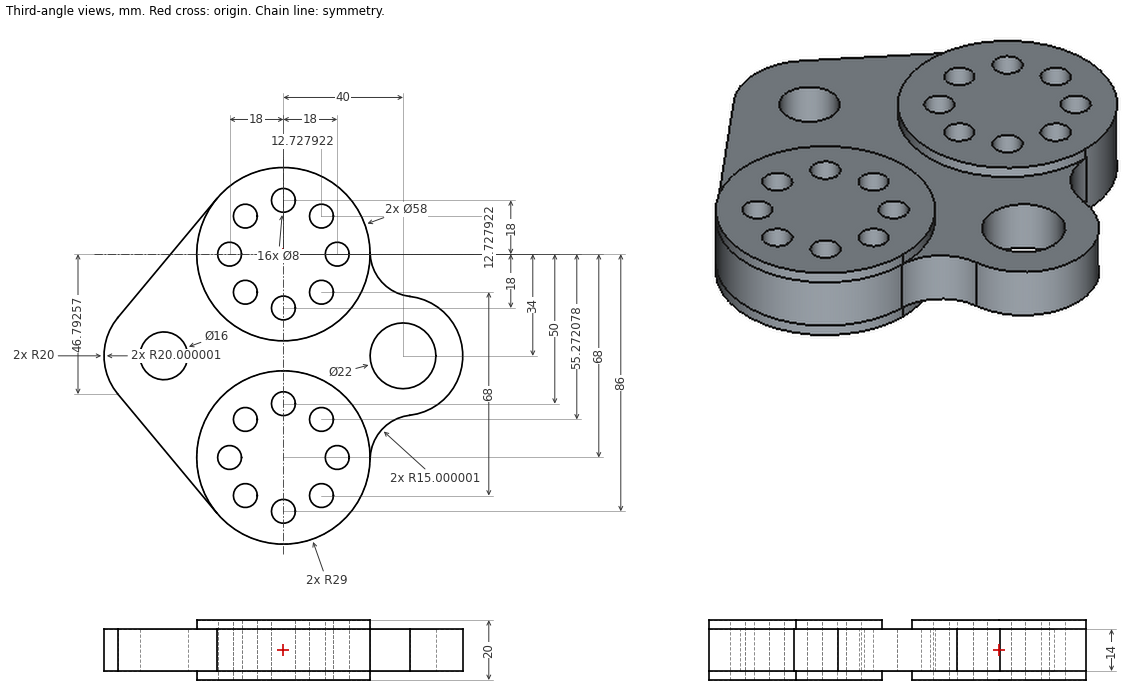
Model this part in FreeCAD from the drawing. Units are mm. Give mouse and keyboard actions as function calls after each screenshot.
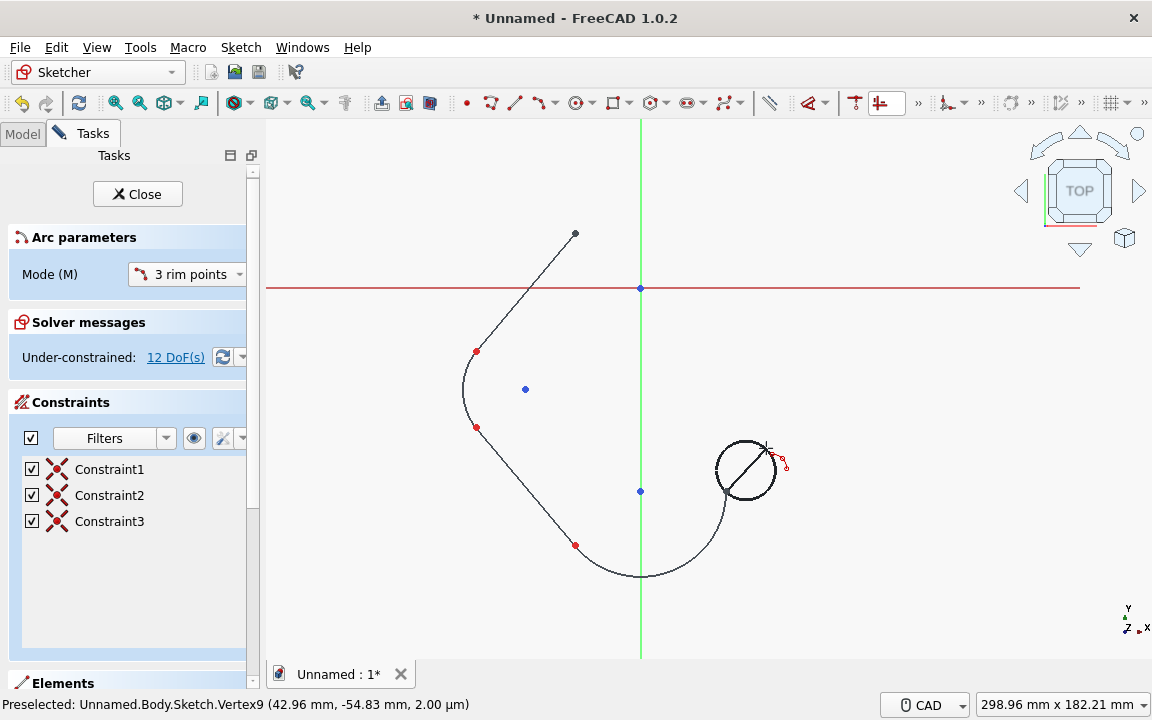
scroll(738, 462, up, 2)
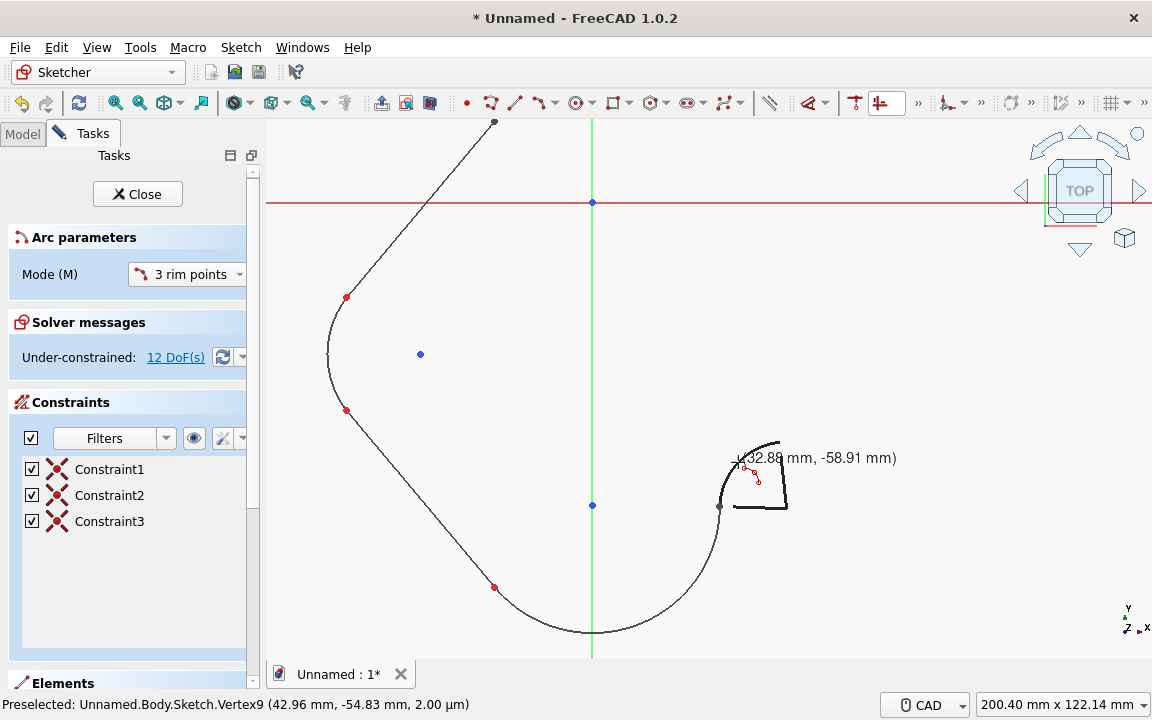
click(738, 462)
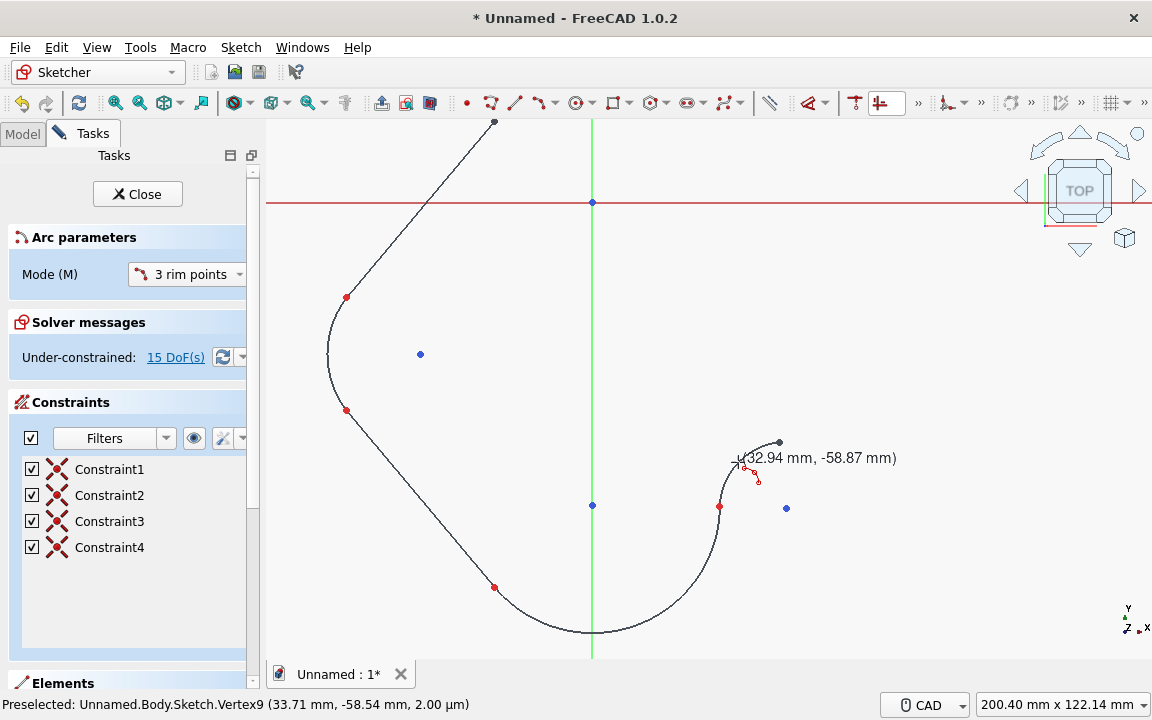
click(780, 442)
click(779, 265)
click(858, 353)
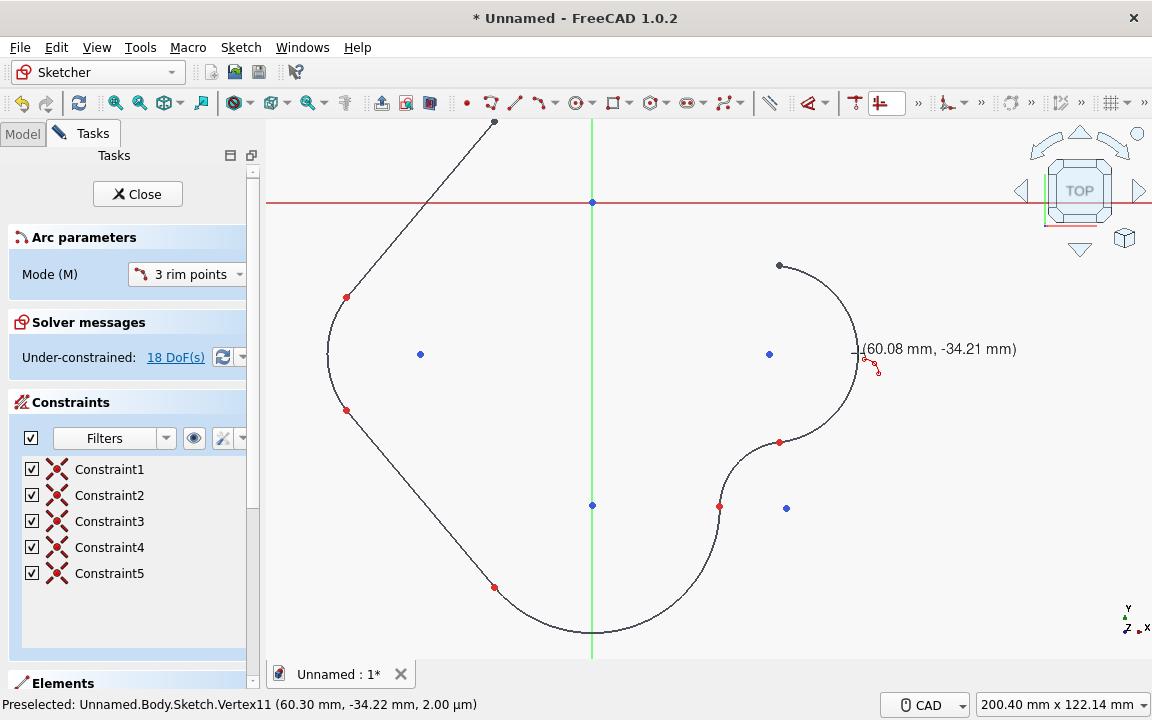
click(779, 266)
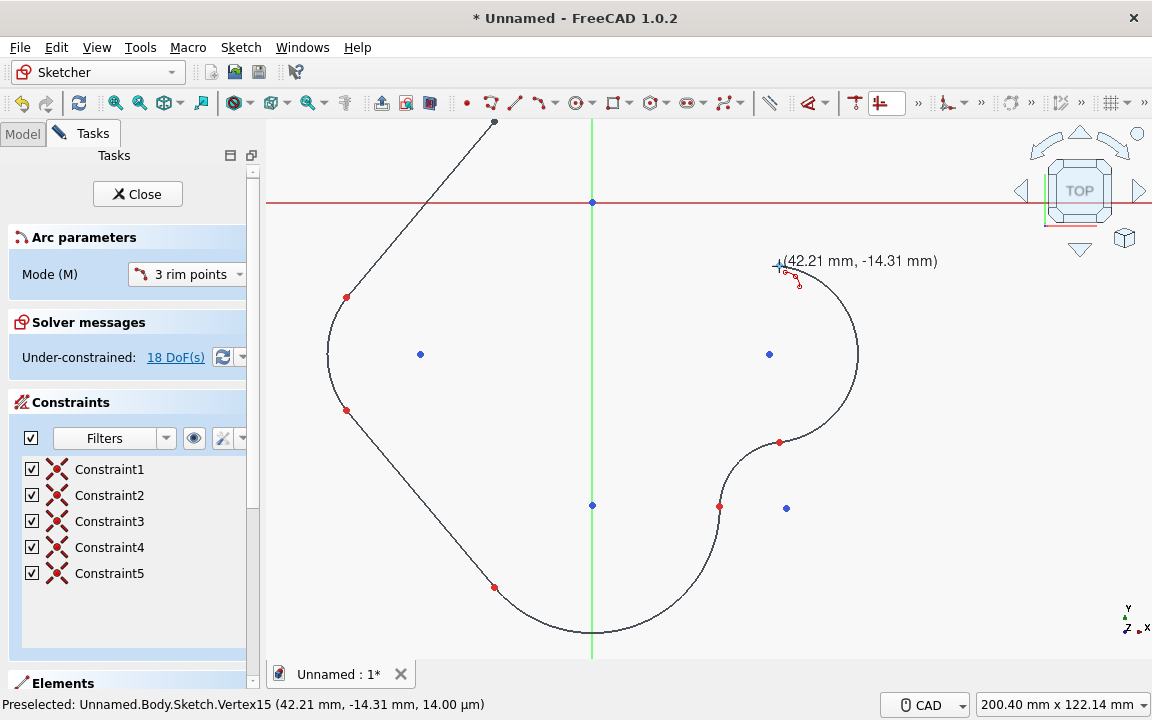
scroll(721, 200, up, 10)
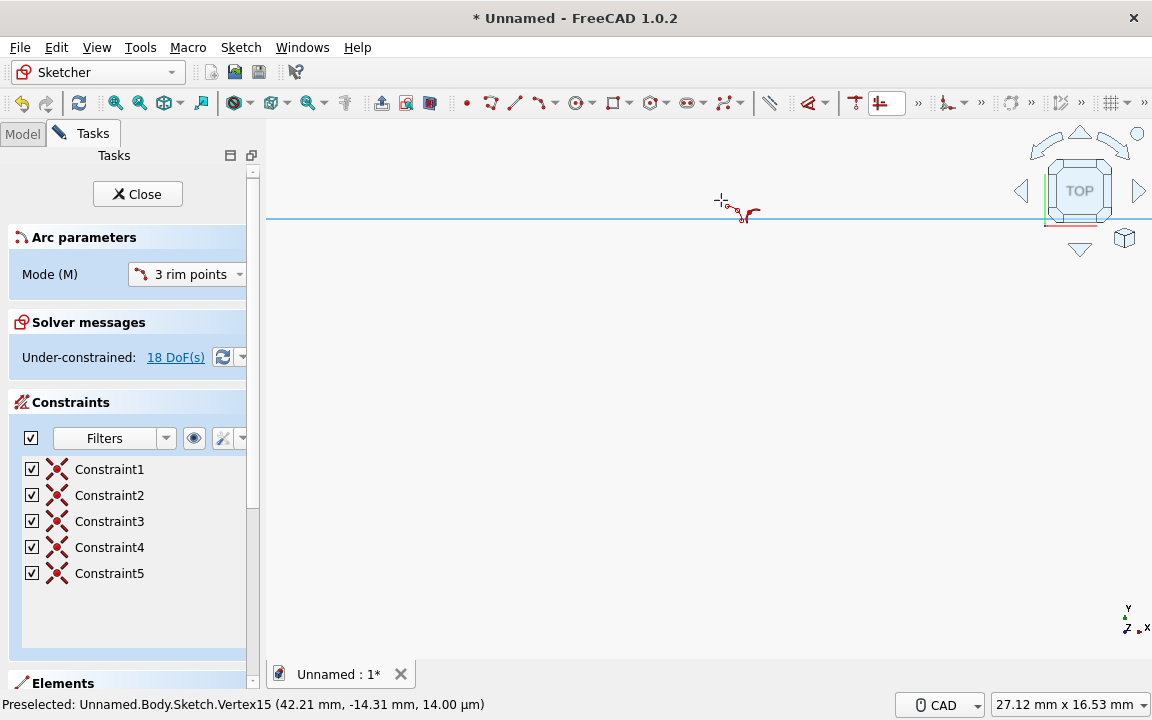
click(715, 203)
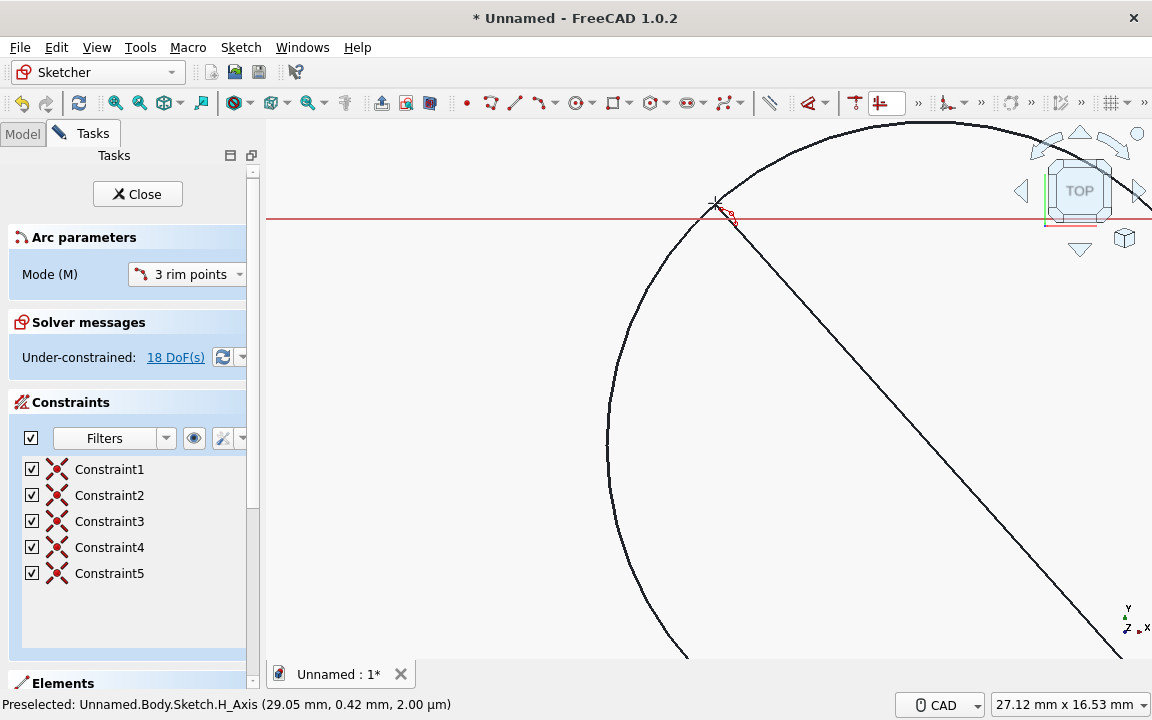
scroll(728, 295, down, 12)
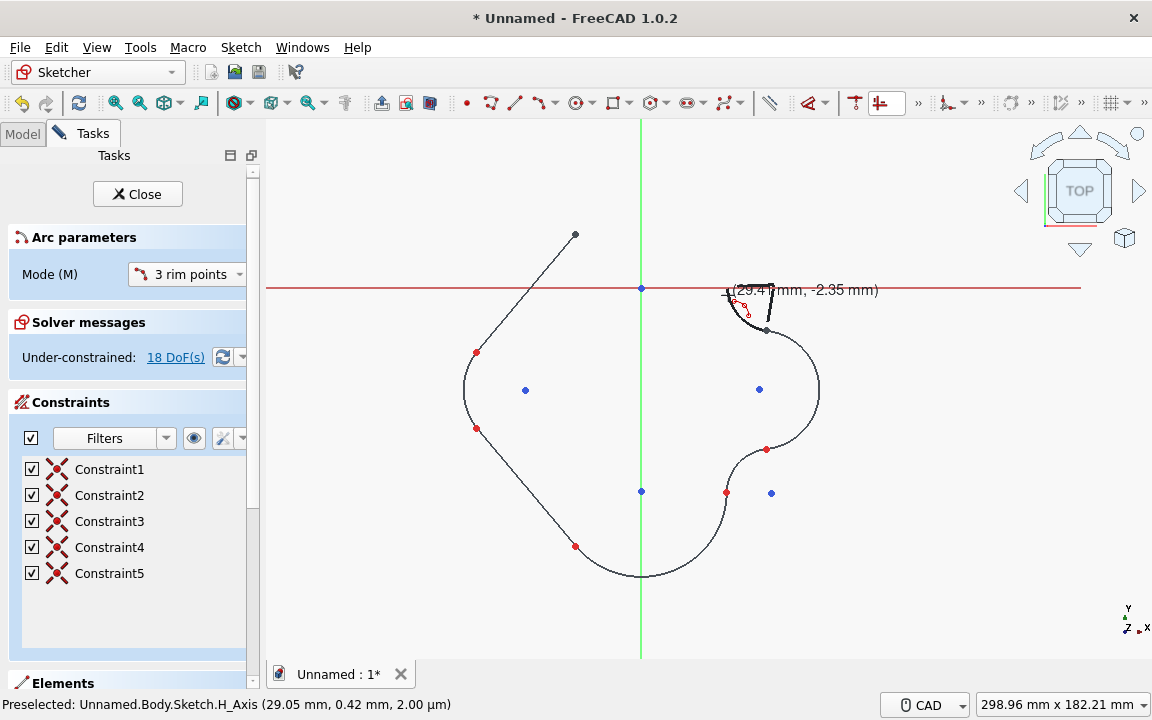
scroll(739, 316, up, 2)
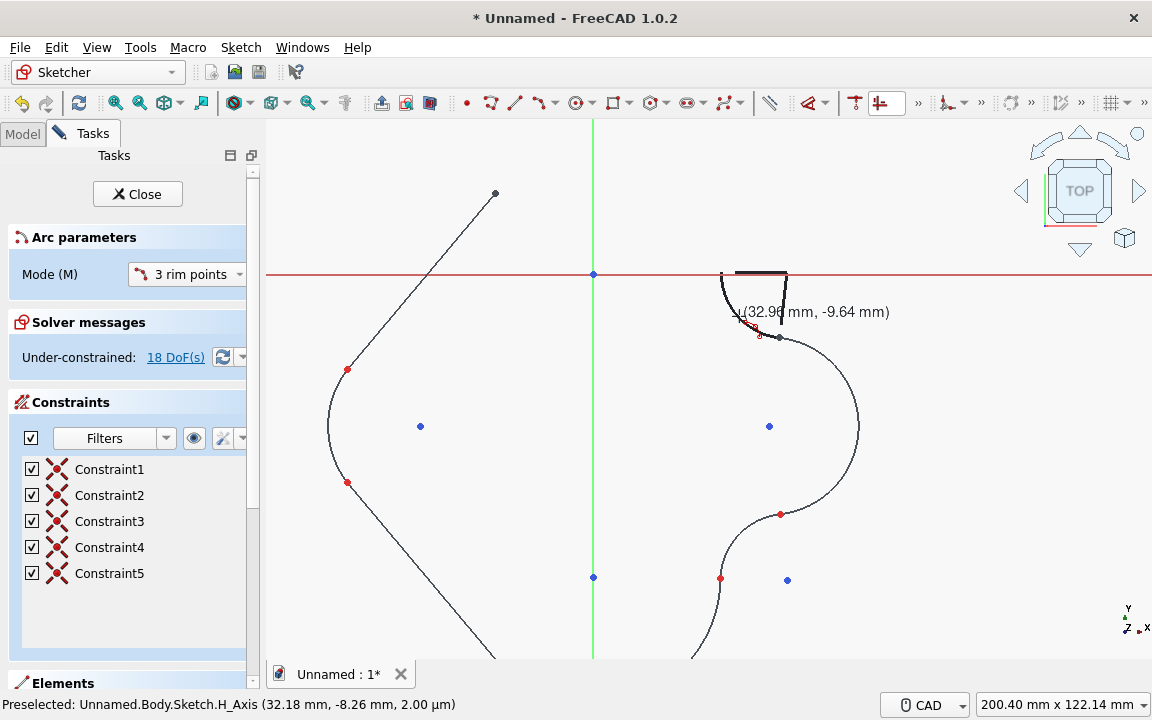
click(738, 316)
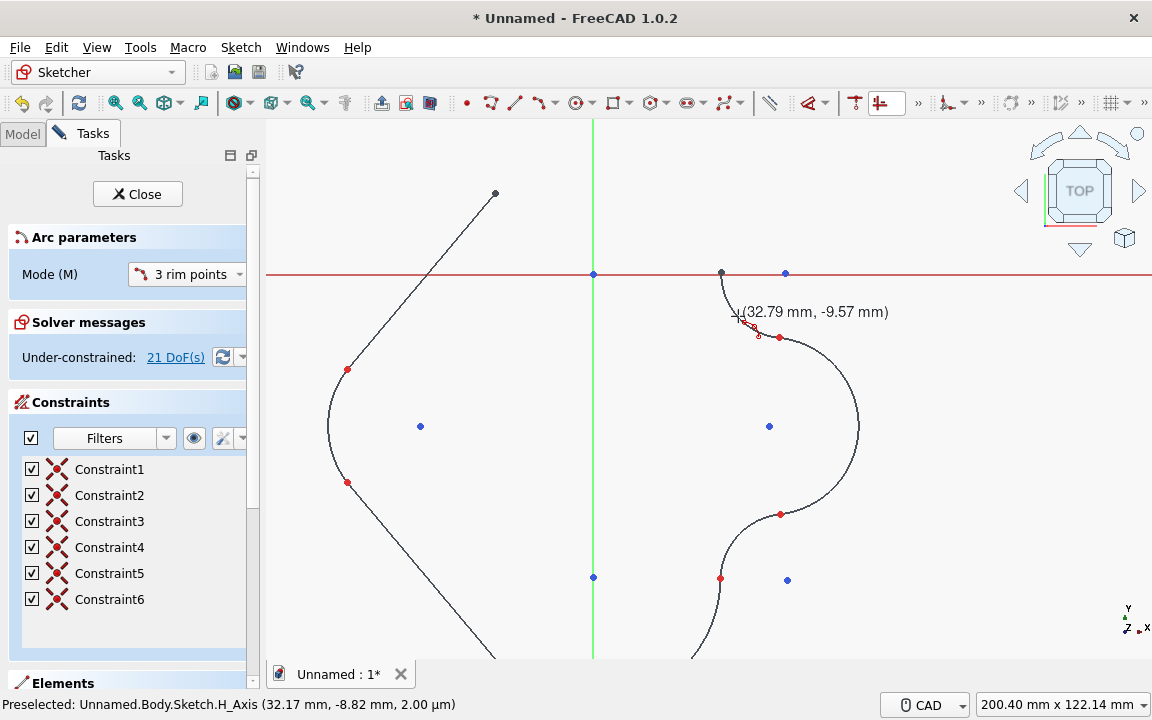
scroll(721, 272, up, 10)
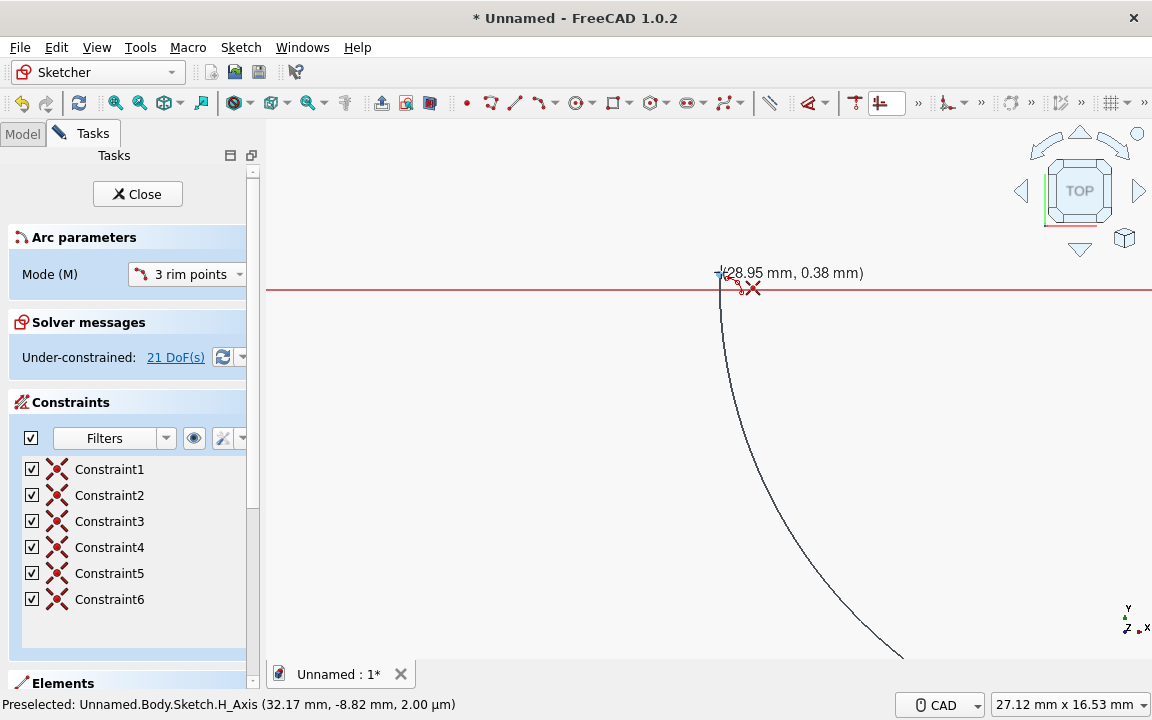
click(720, 275)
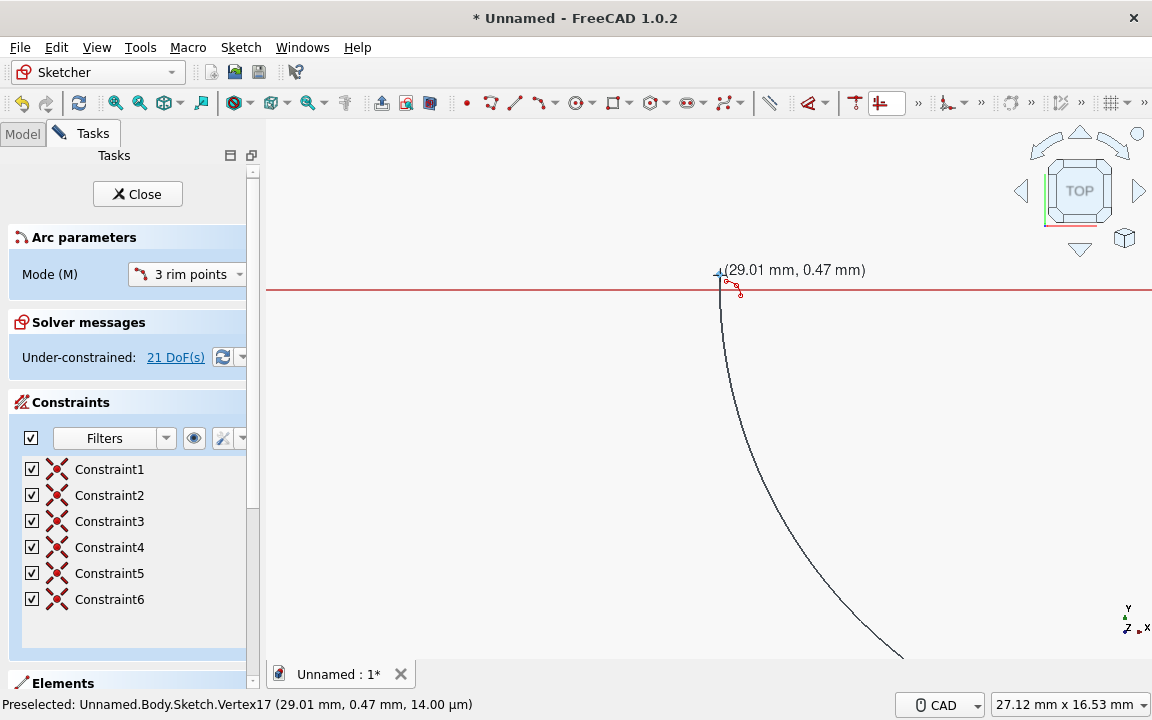
scroll(727, 288, down, 12)